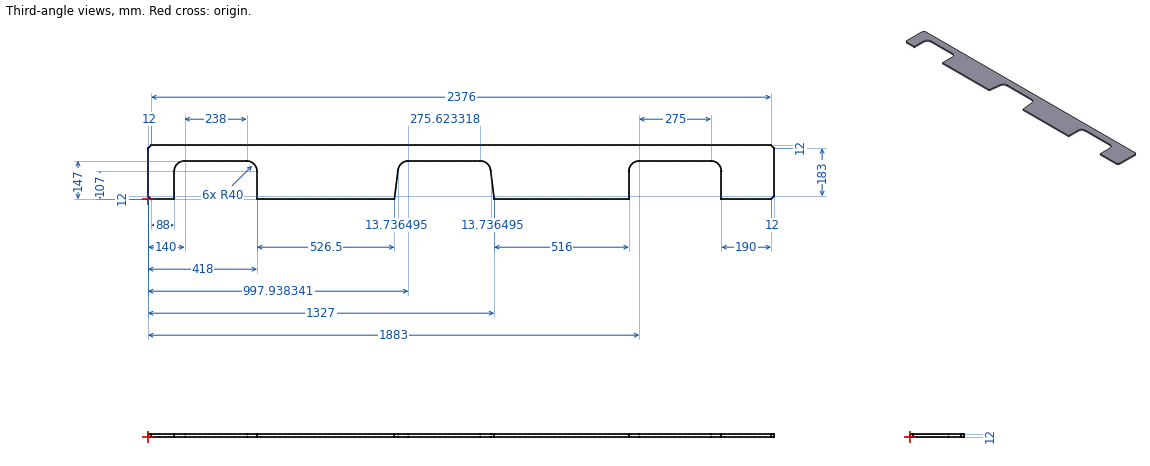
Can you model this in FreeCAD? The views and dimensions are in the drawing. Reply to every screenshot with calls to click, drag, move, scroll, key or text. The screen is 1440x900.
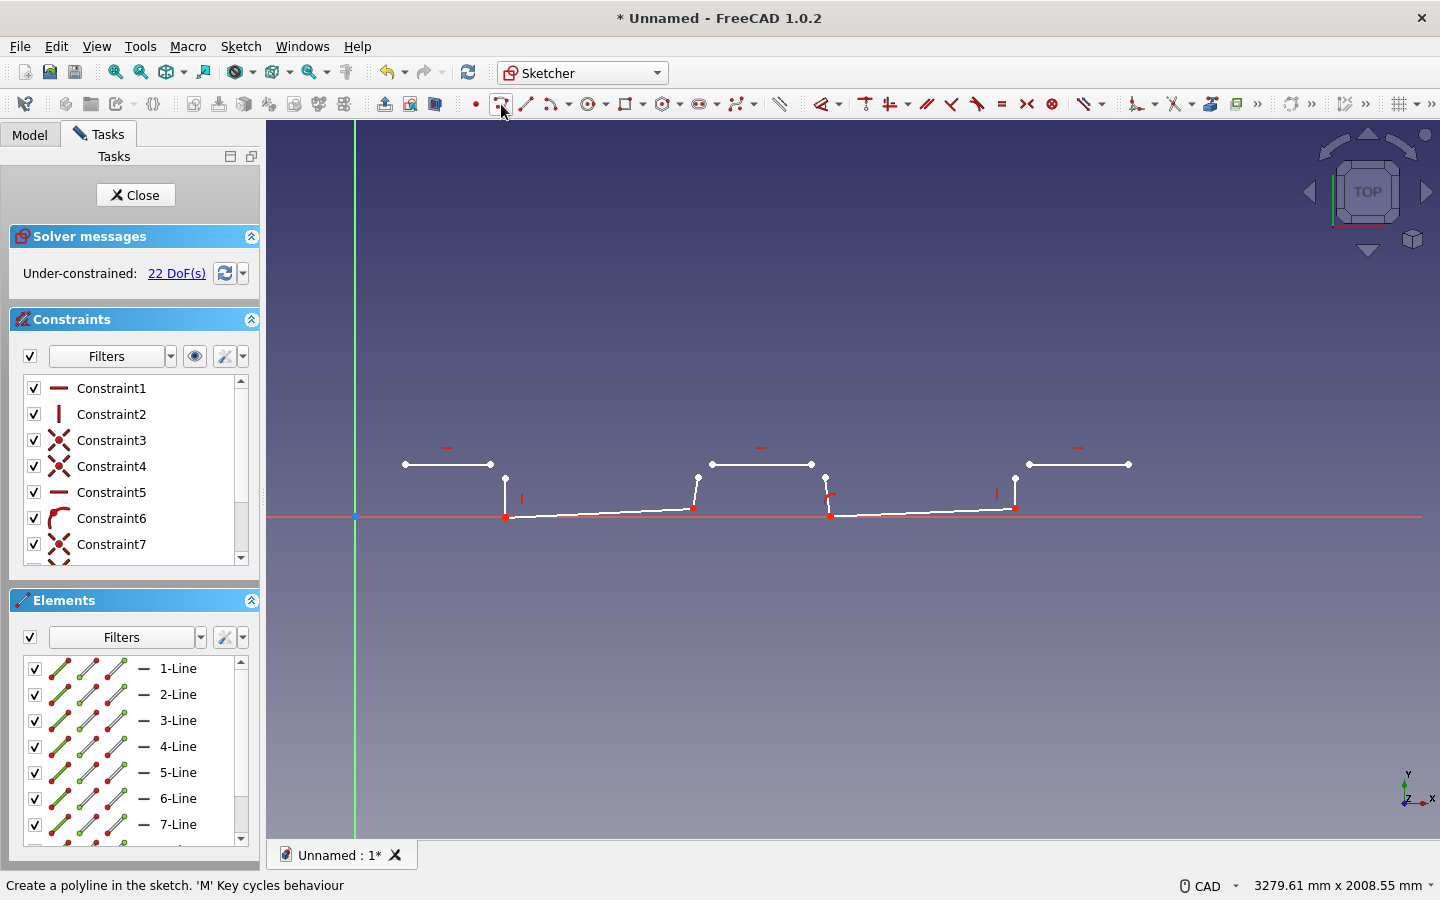
click(1142, 478)
click(1142, 517)
click(1210, 508)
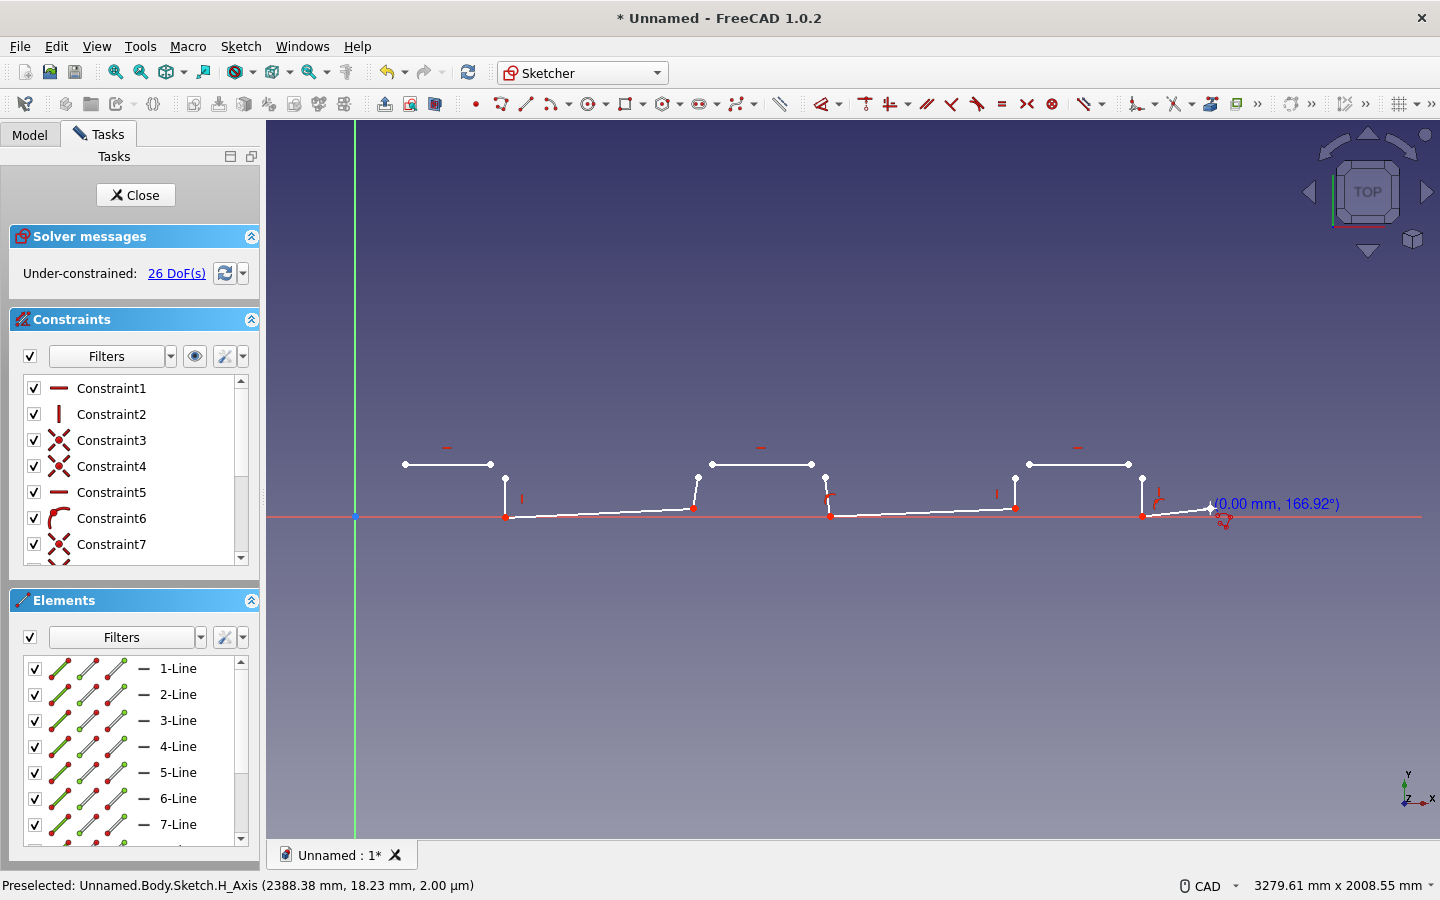
scroll(1214, 512, up, 7)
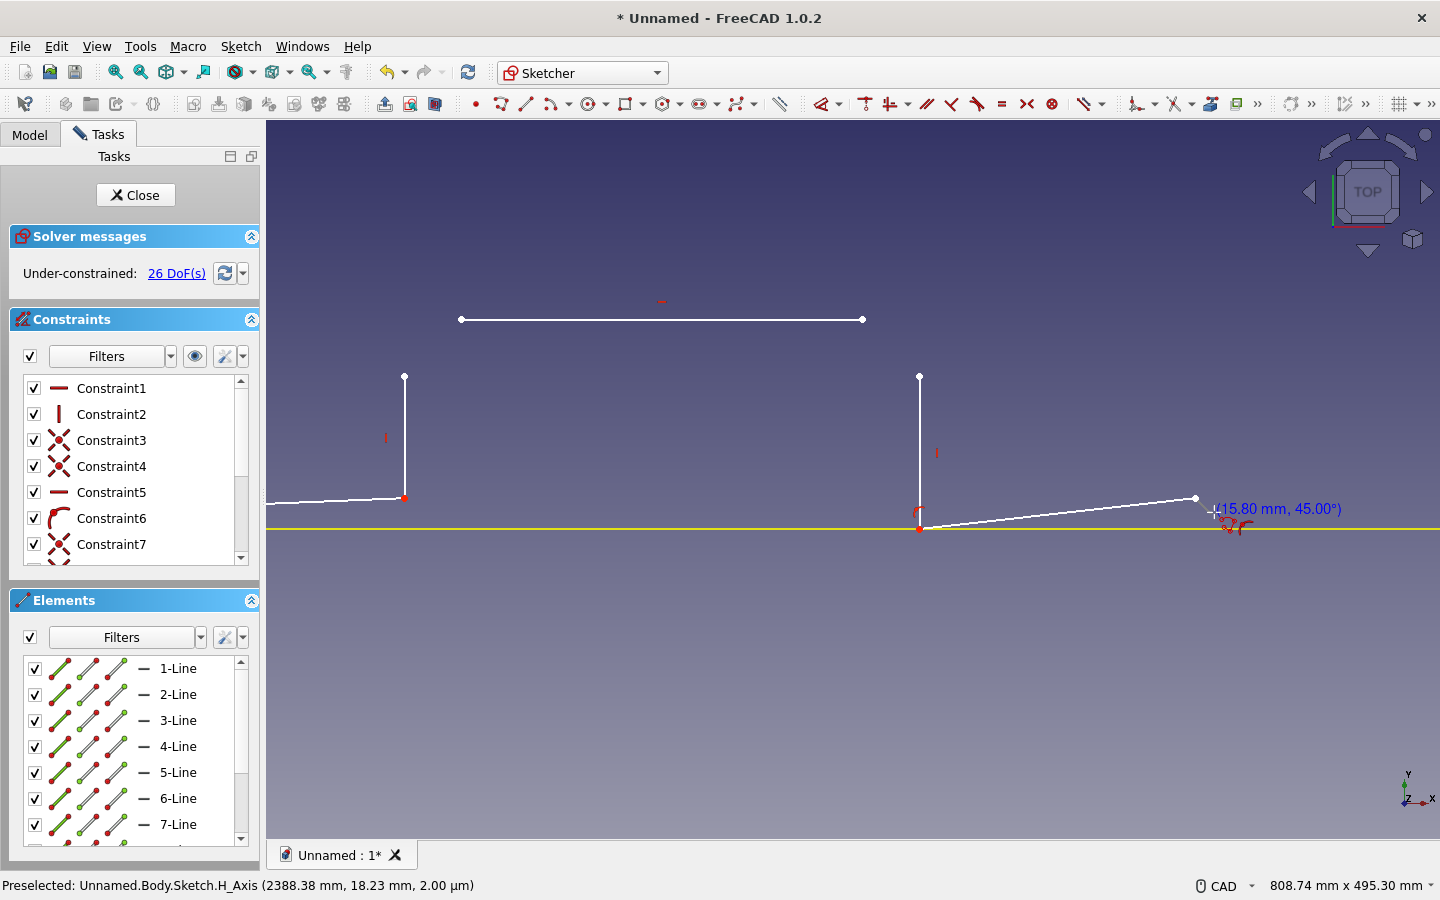
click(1213, 512)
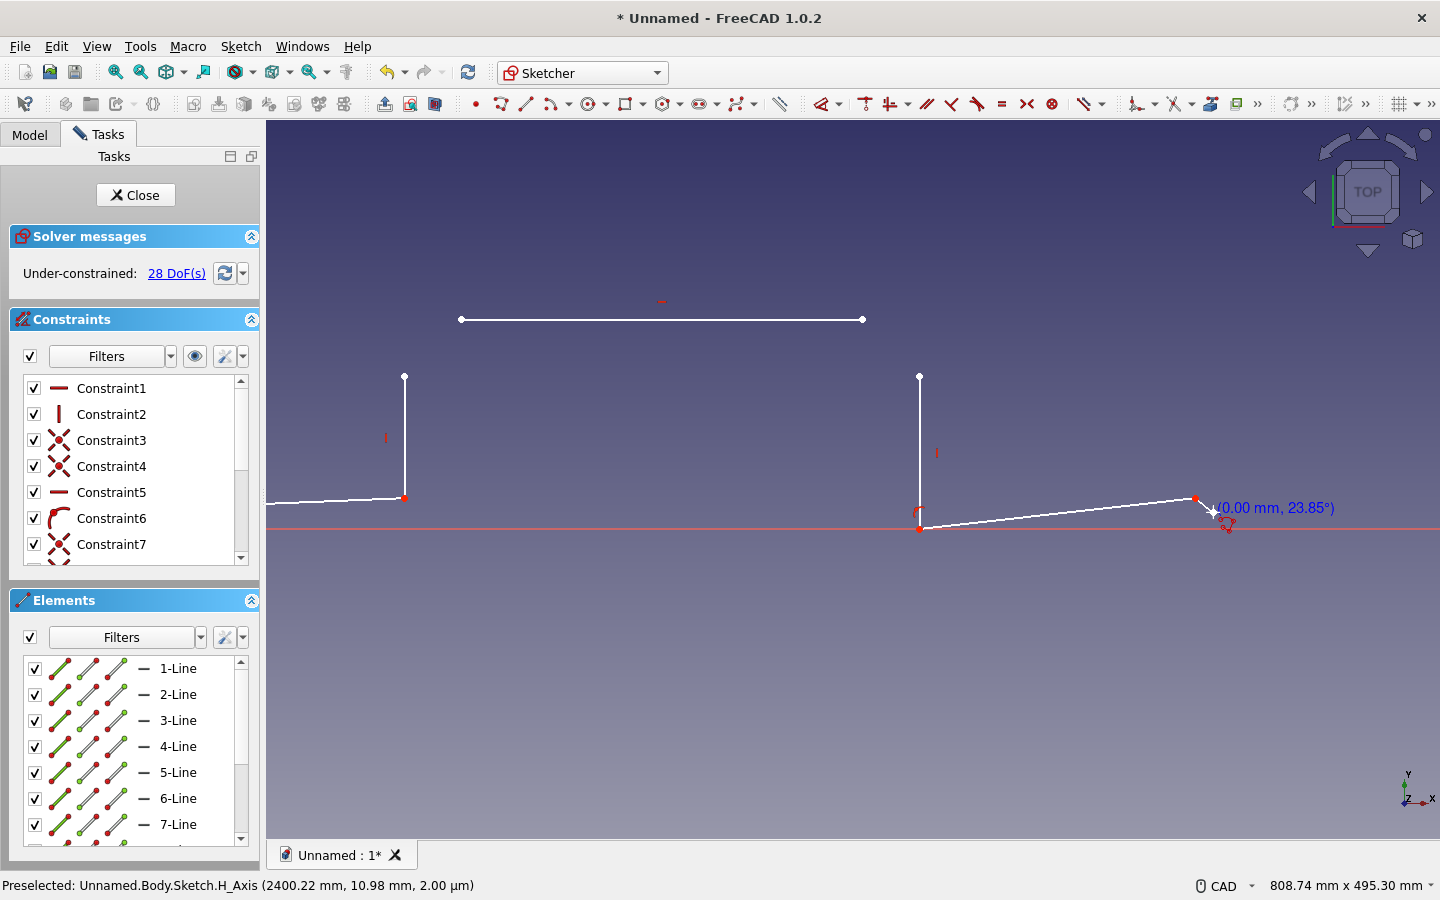
scroll(1117, 505, down, 8)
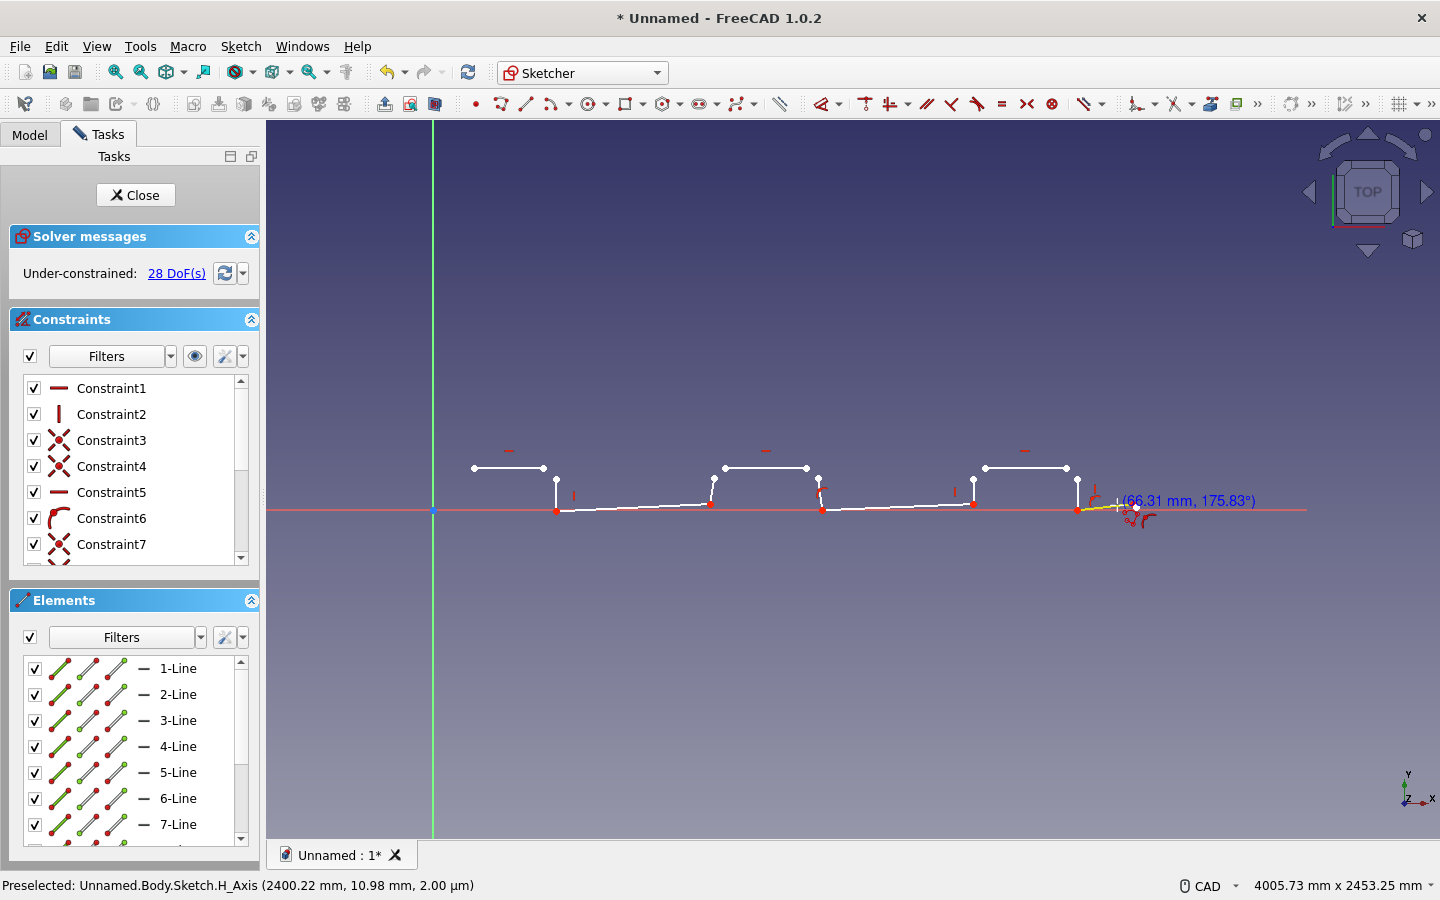
click(1137, 453)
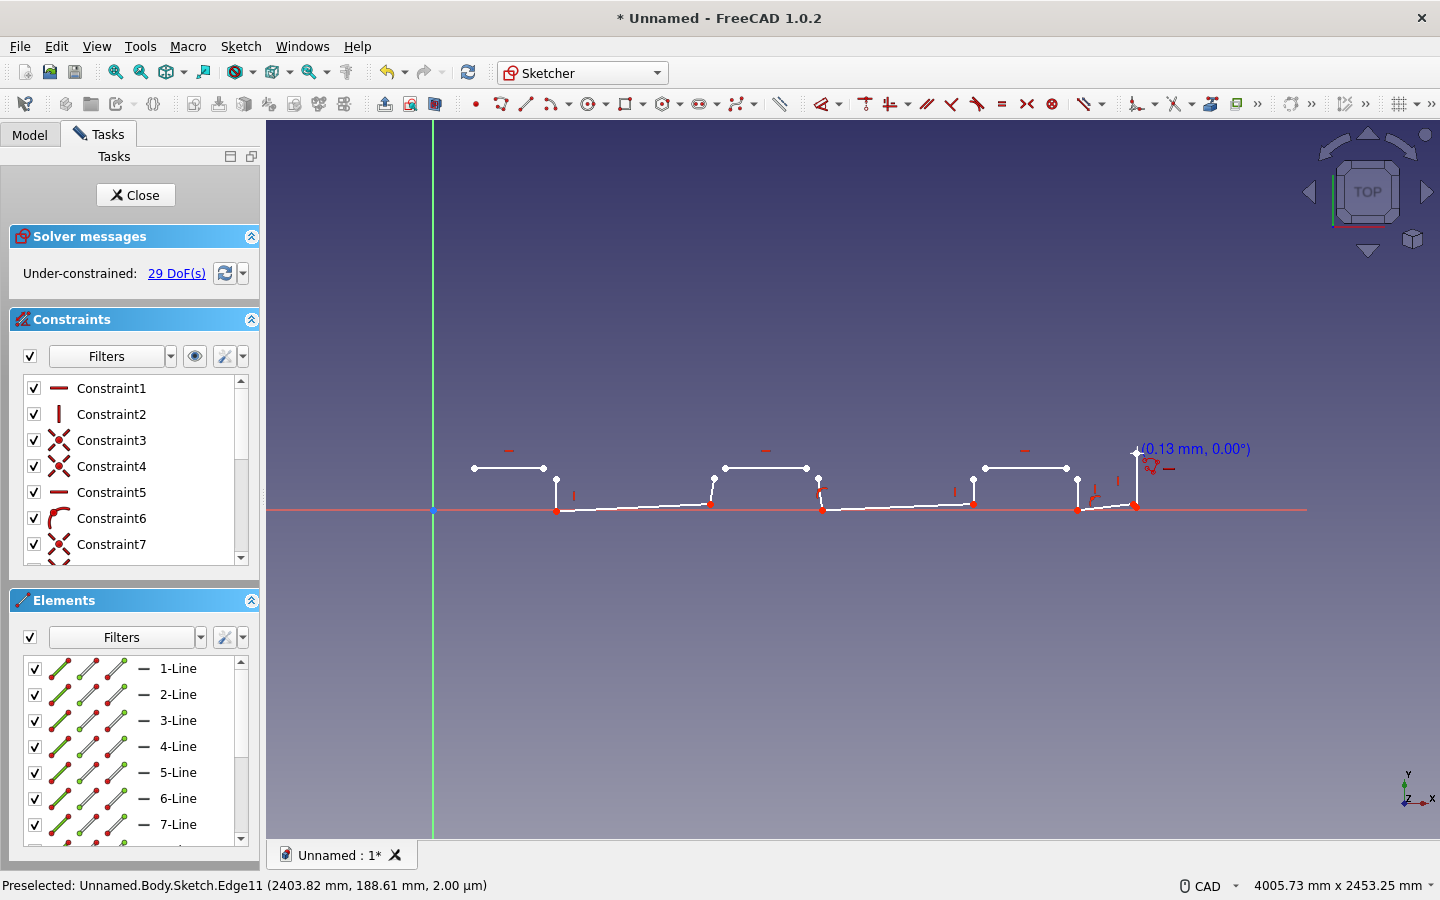
scroll(1133, 450, up, 6)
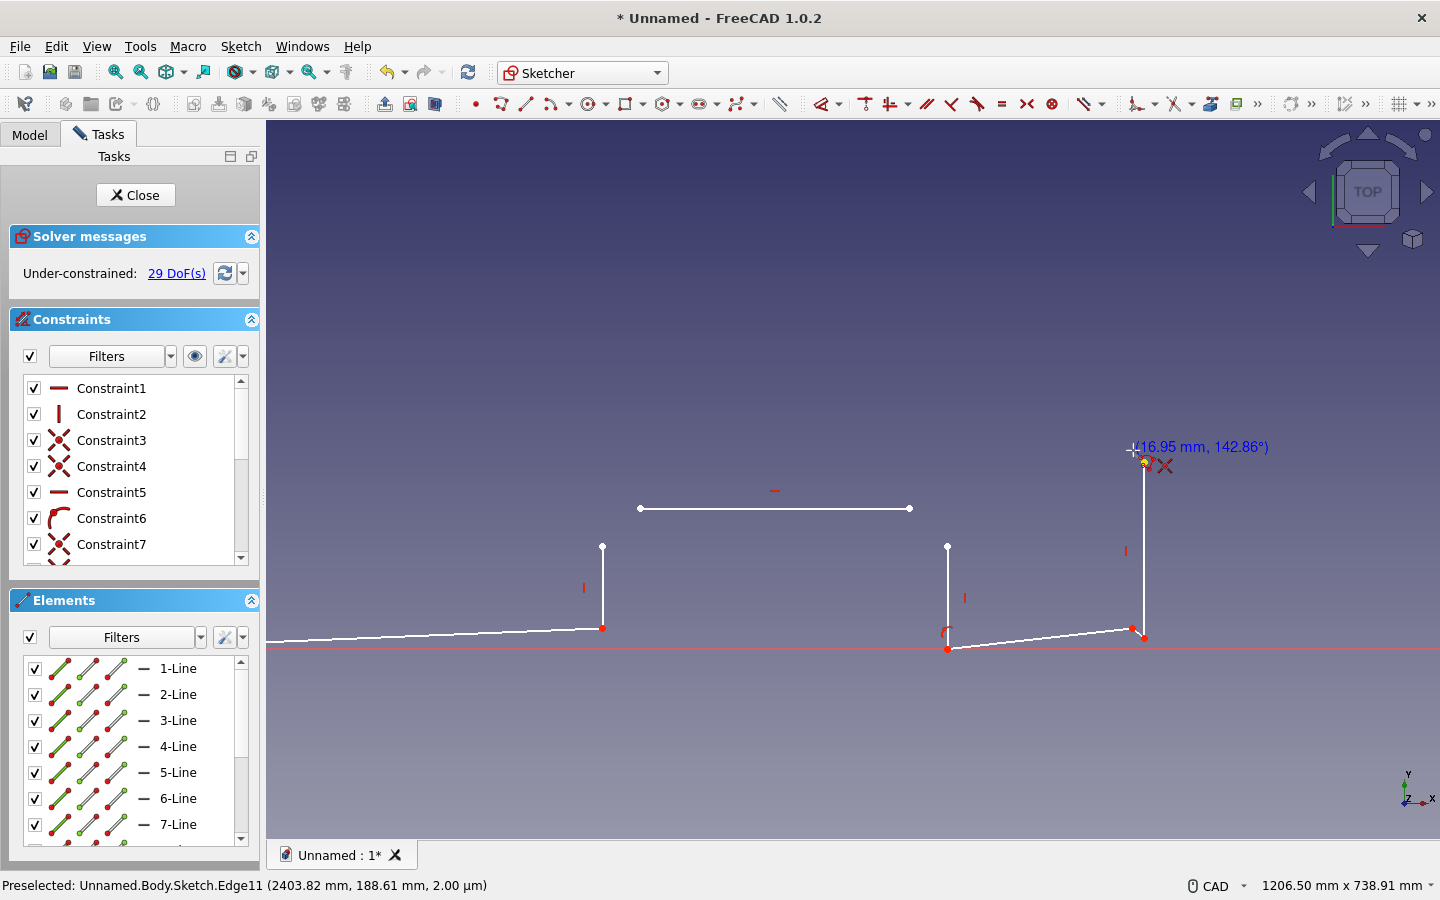
click(1132, 448)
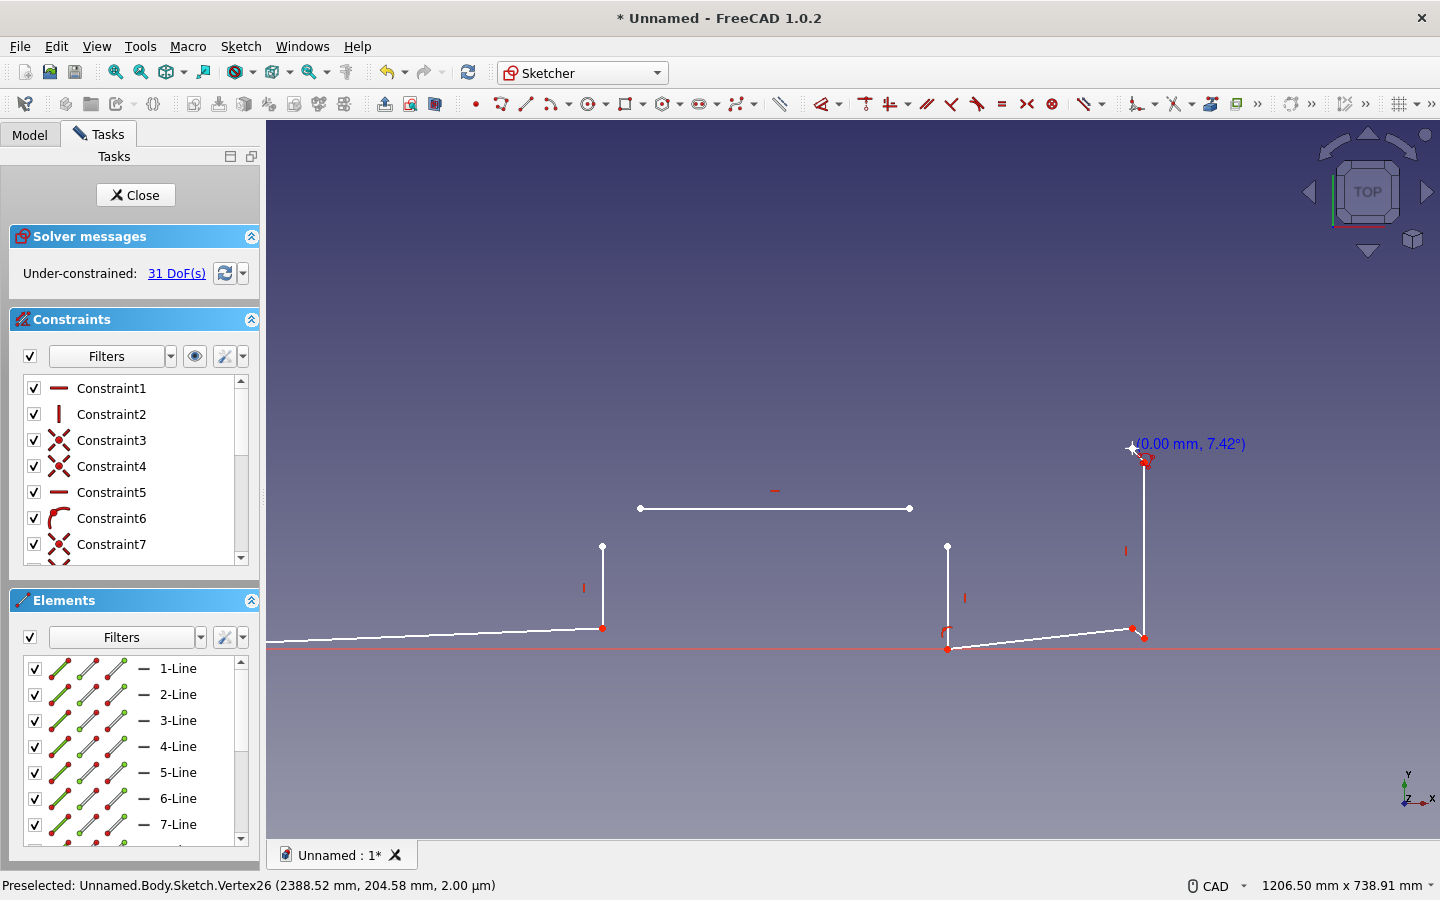
scroll(1133, 450, down, 6)